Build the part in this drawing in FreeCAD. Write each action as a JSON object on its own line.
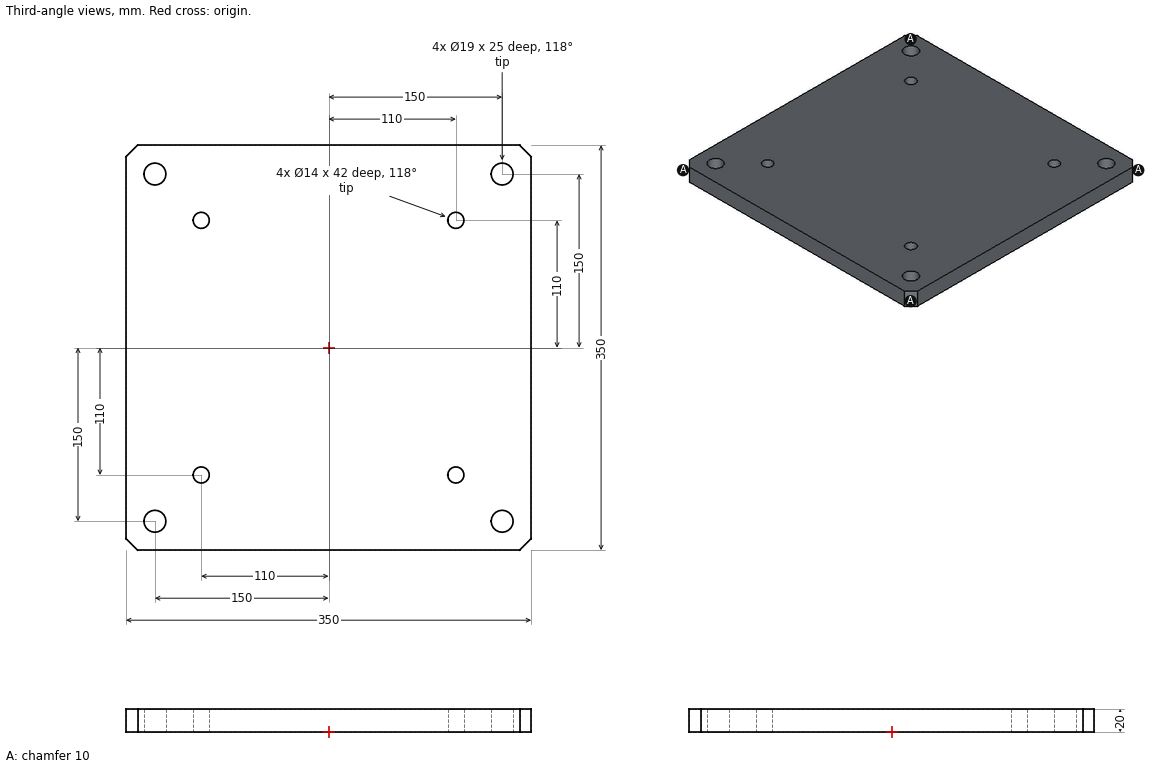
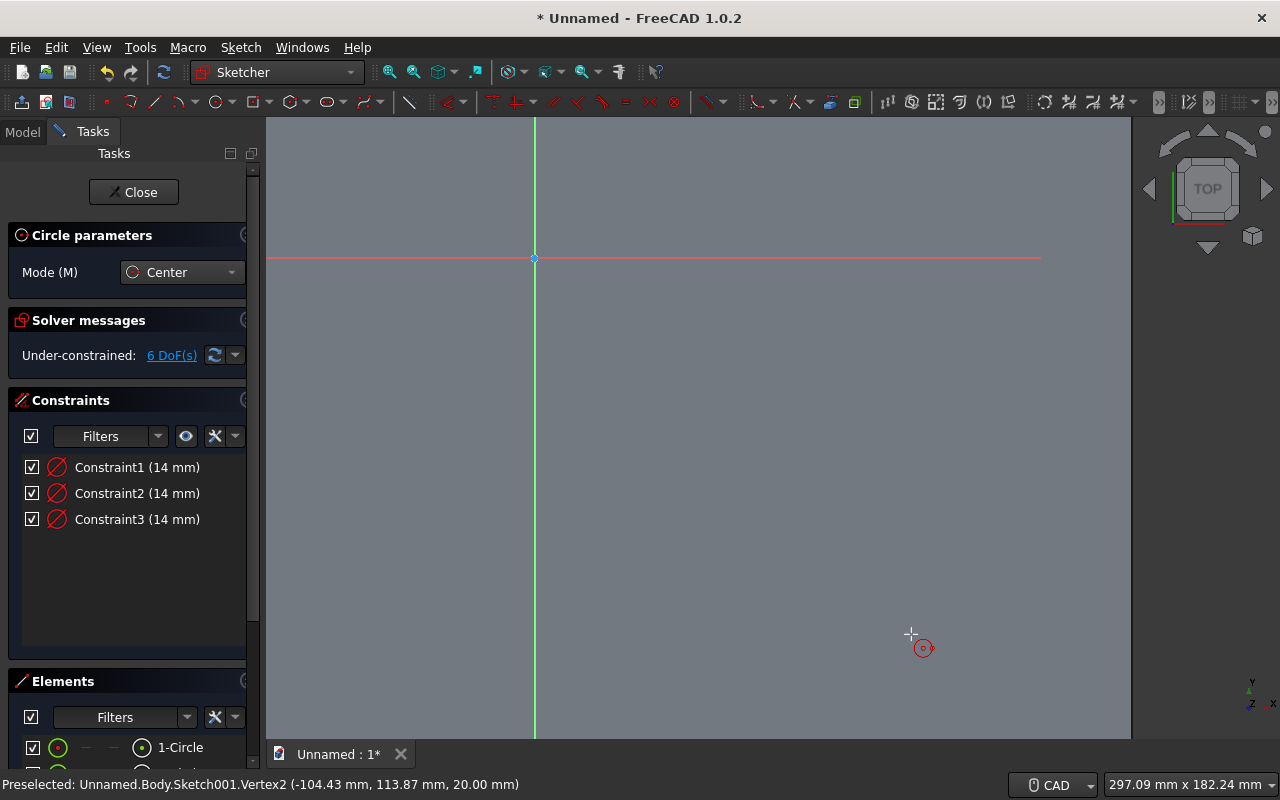
{"action": "left_click", "coordinate": [910, 634]}
{"action": "mouse_move", "coordinate": [927, 617]}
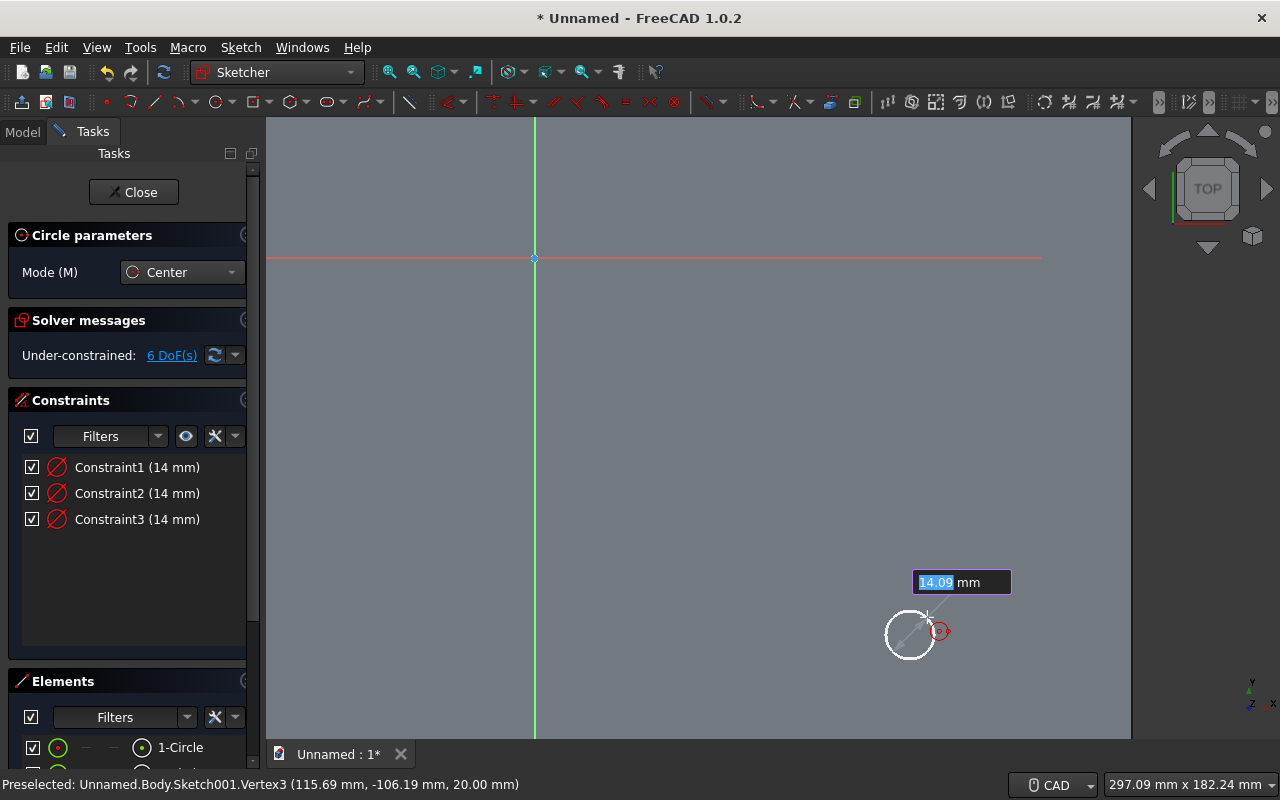
{"action": "type", "text": "14"}
{"action": "key", "text": "Return"}
{"action": "key", "text": "Escape"}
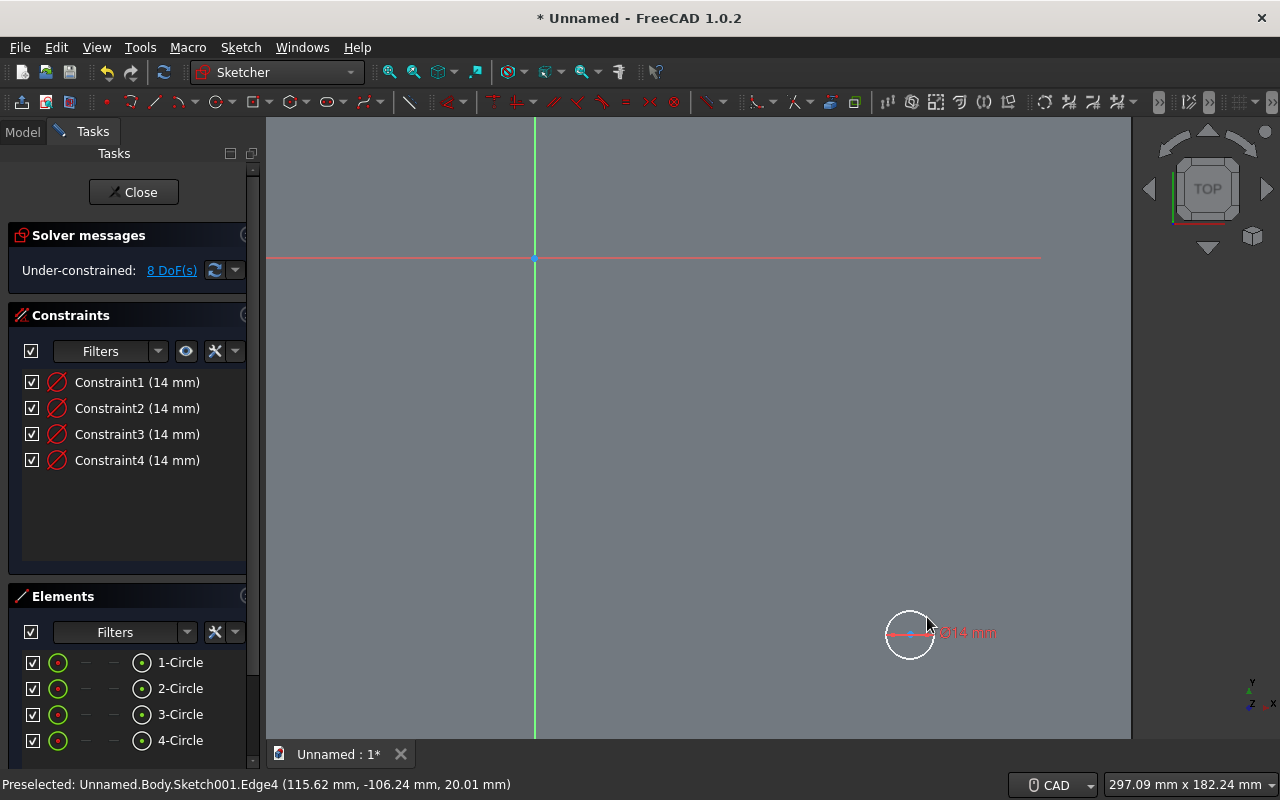
{"action": "scroll", "coordinate": [911, 634], "scroll_direction": "down", "scroll_amount": 3}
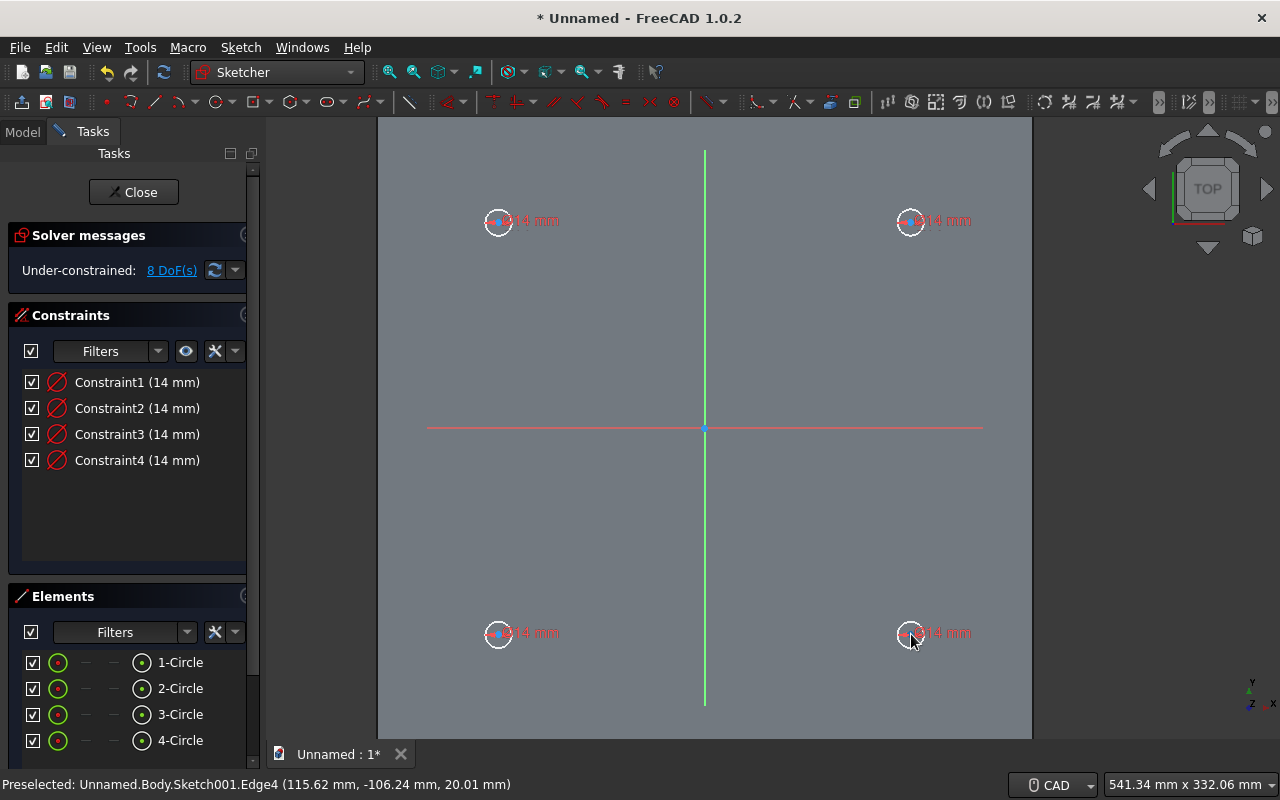
{"action": "left_click", "coordinate": [499, 635]}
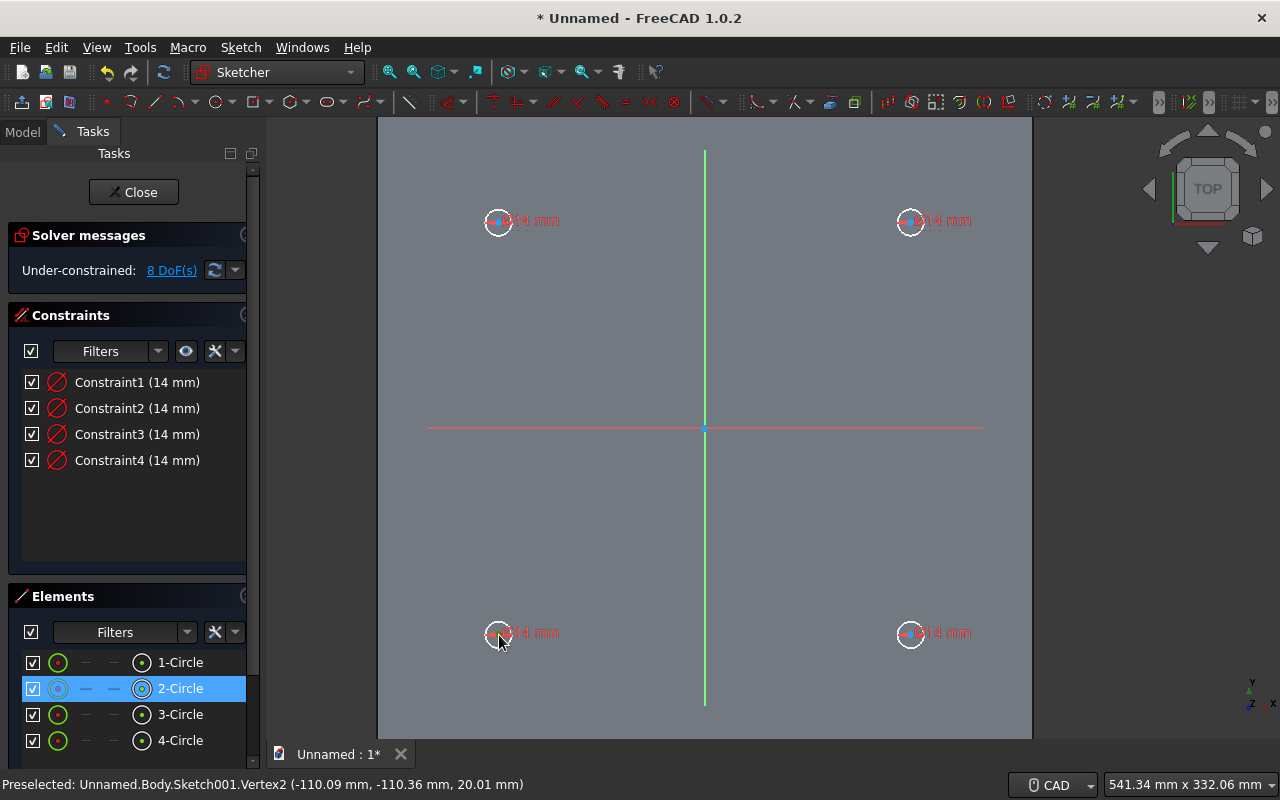
{"action": "left_click", "coordinate": [499, 223]}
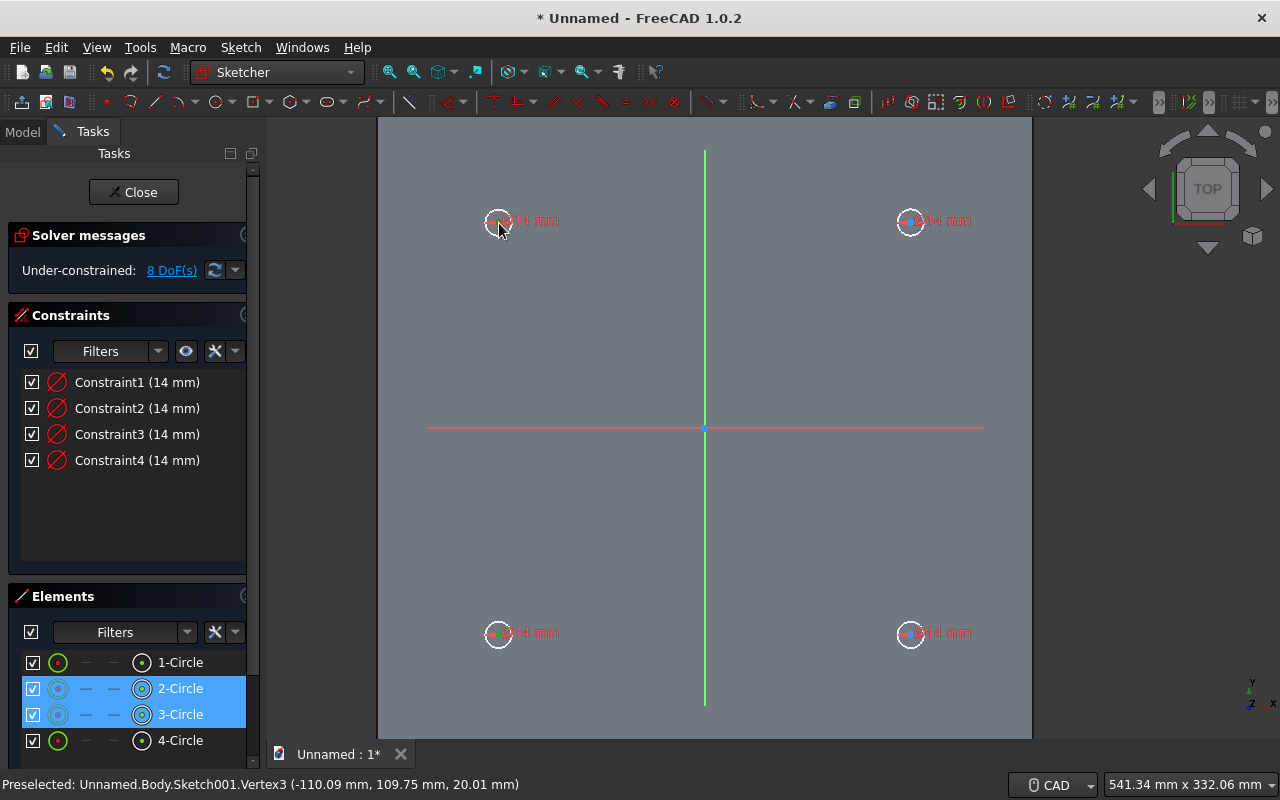
{"action": "left_click", "coordinate": [536, 102]}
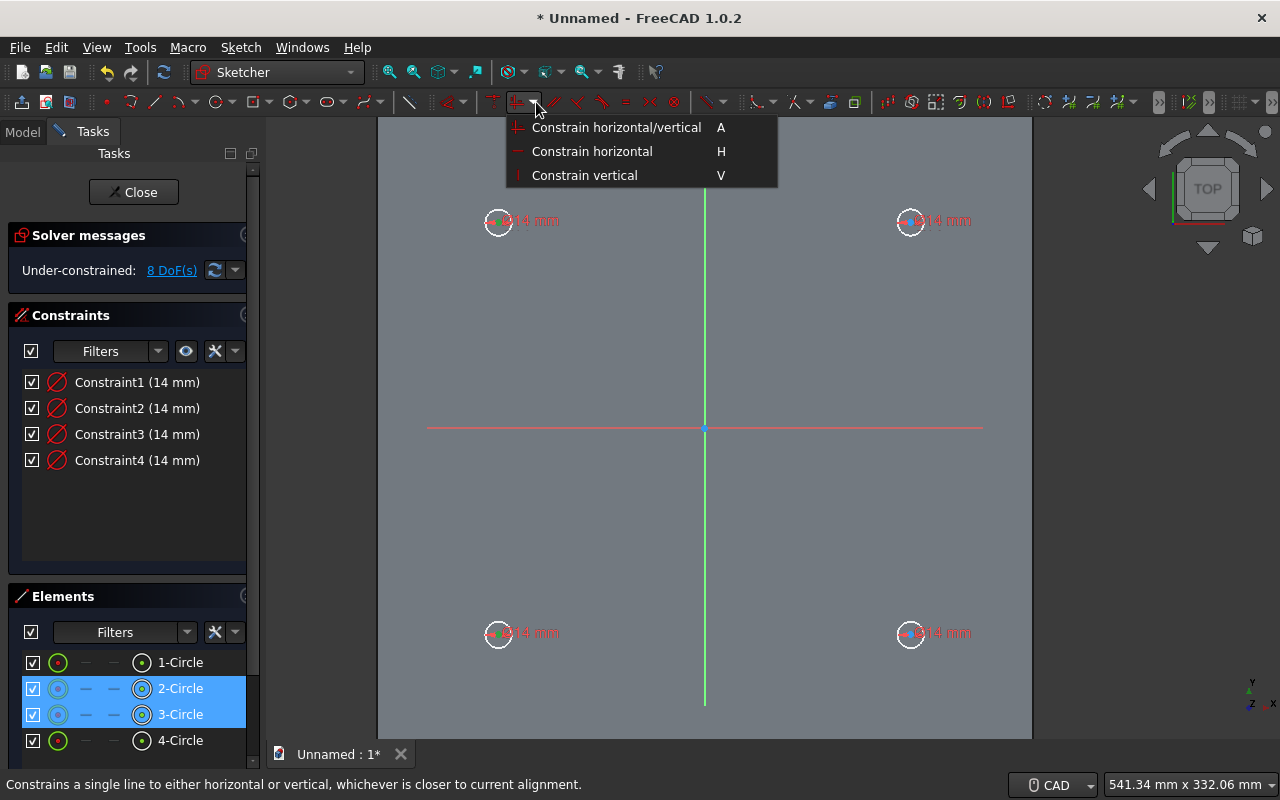
{"action": "left_click", "coordinate": [642, 175]}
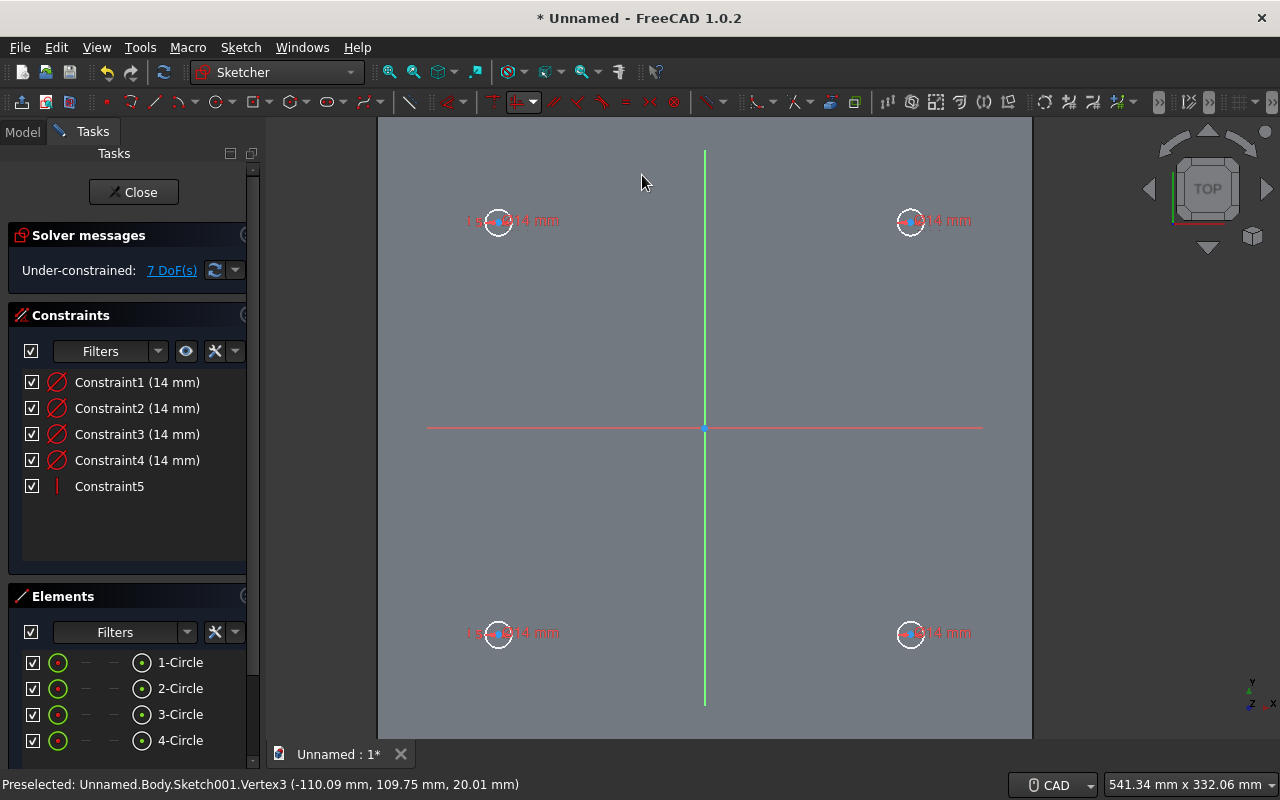
{"action": "left_click", "coordinate": [911, 223]}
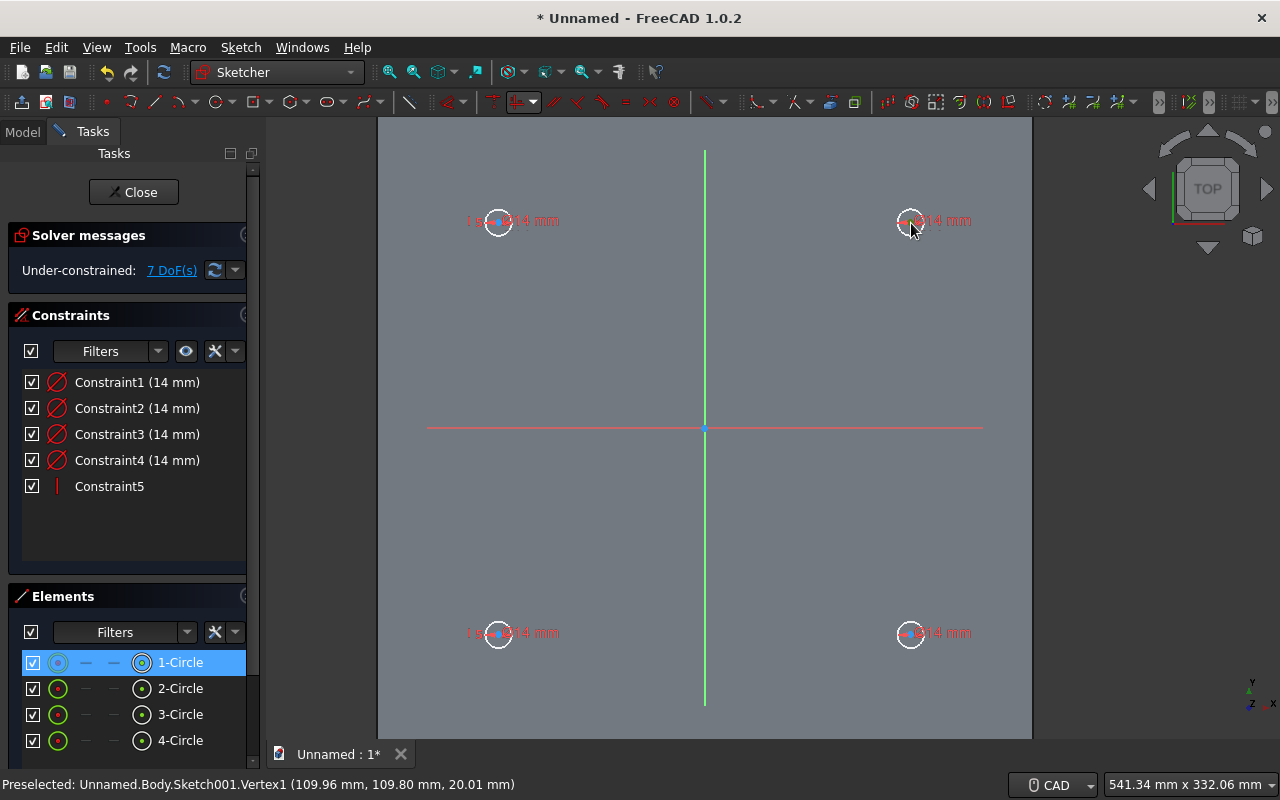
{"action": "left_click", "coordinate": [499, 223]}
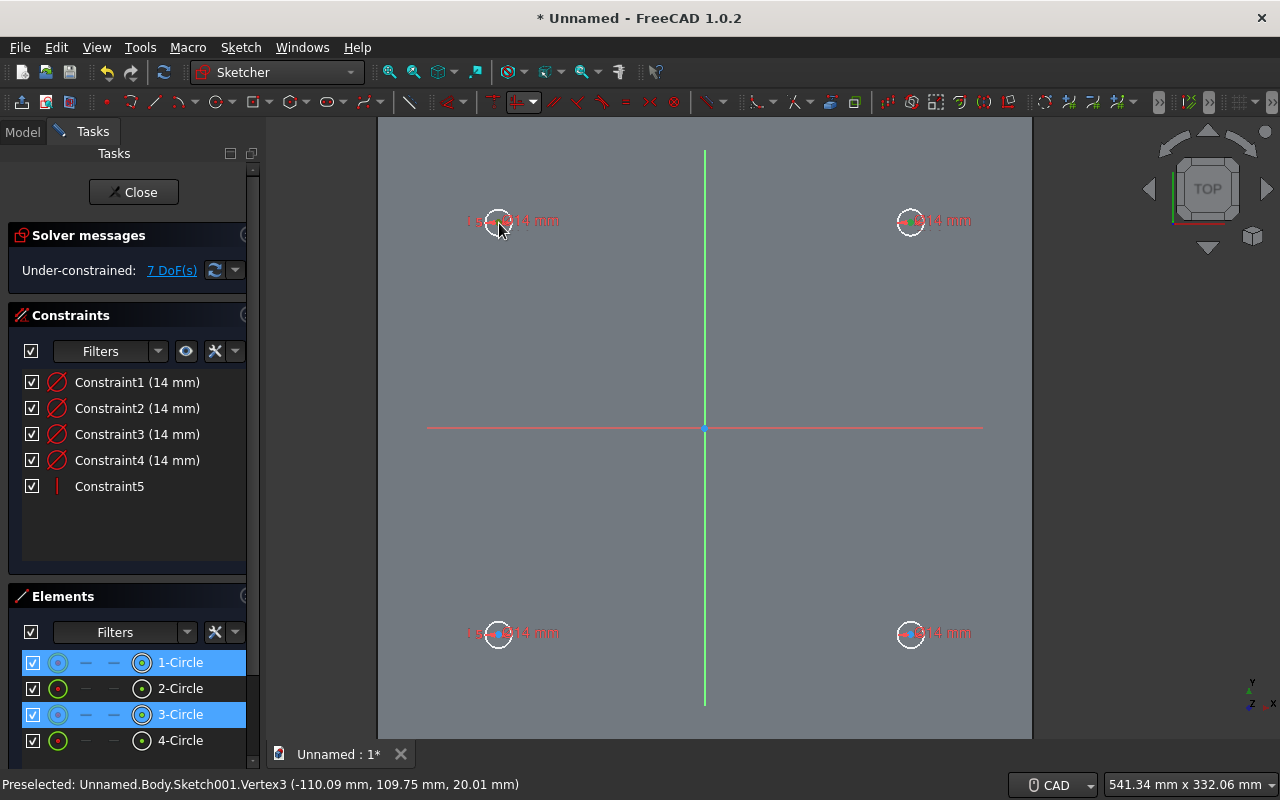
{"action": "left_click", "coordinate": [536, 102]}